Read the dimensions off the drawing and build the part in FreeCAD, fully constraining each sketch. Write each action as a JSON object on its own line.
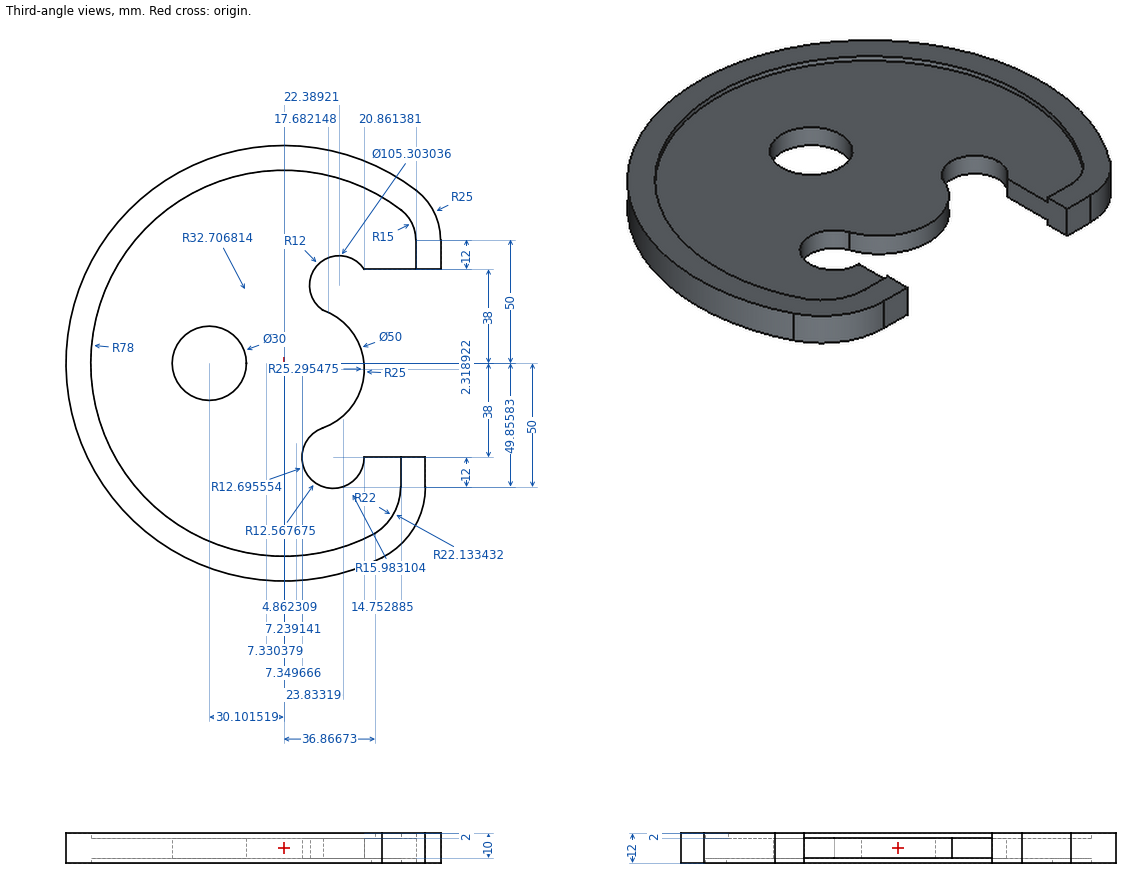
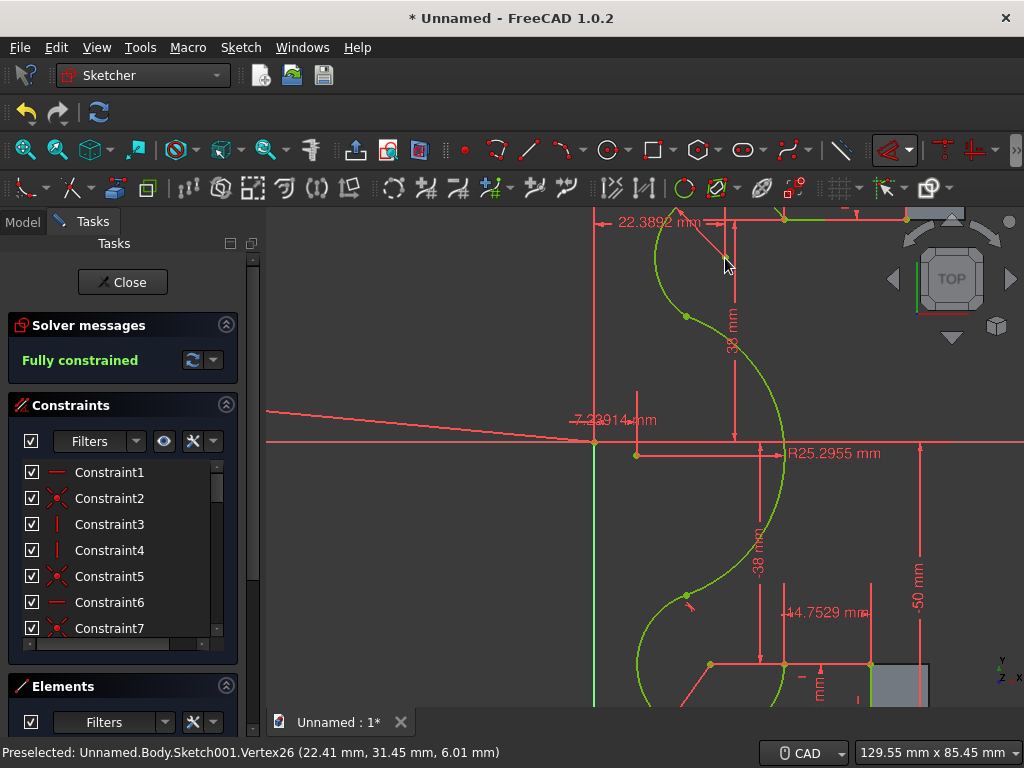
{"action": "left_click", "coordinate": [123, 282]}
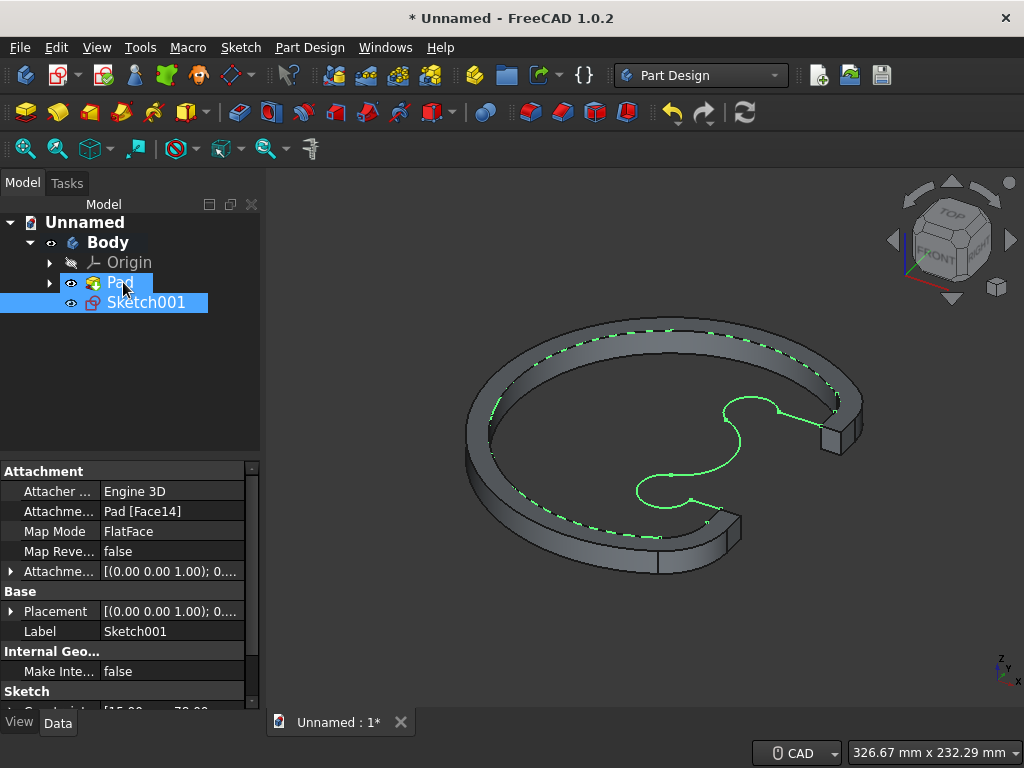
{"action": "left_click", "coordinate": [26, 112]}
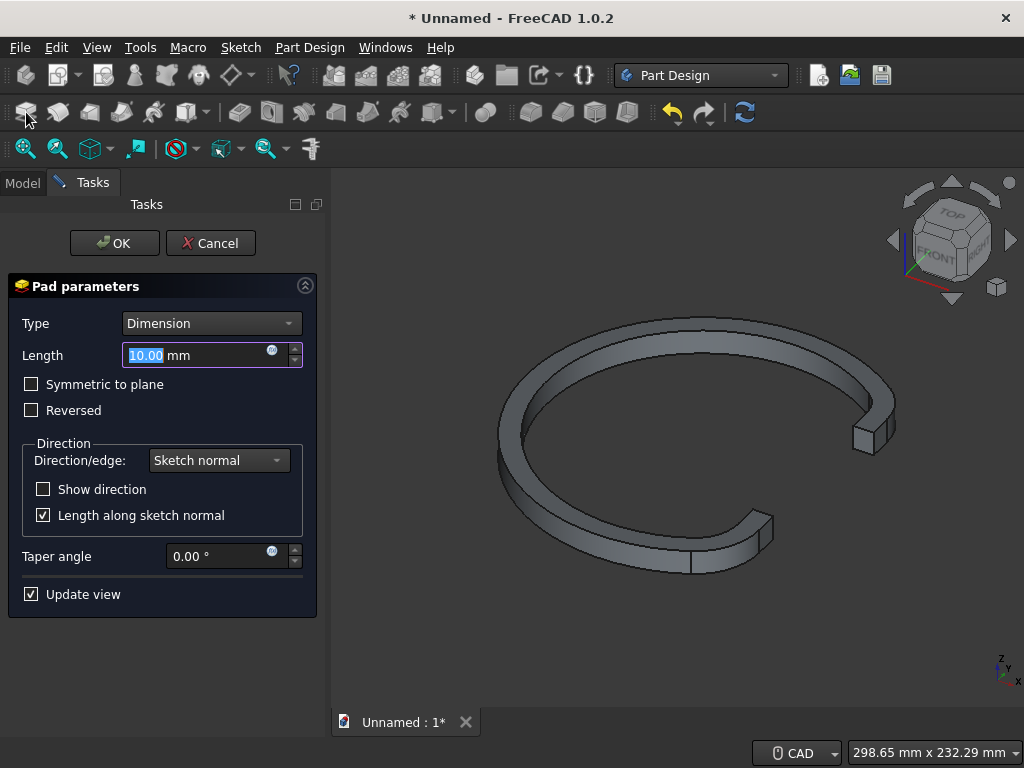
{"action": "type", "text": "10"}
{"action": "key", "text": "Tab"}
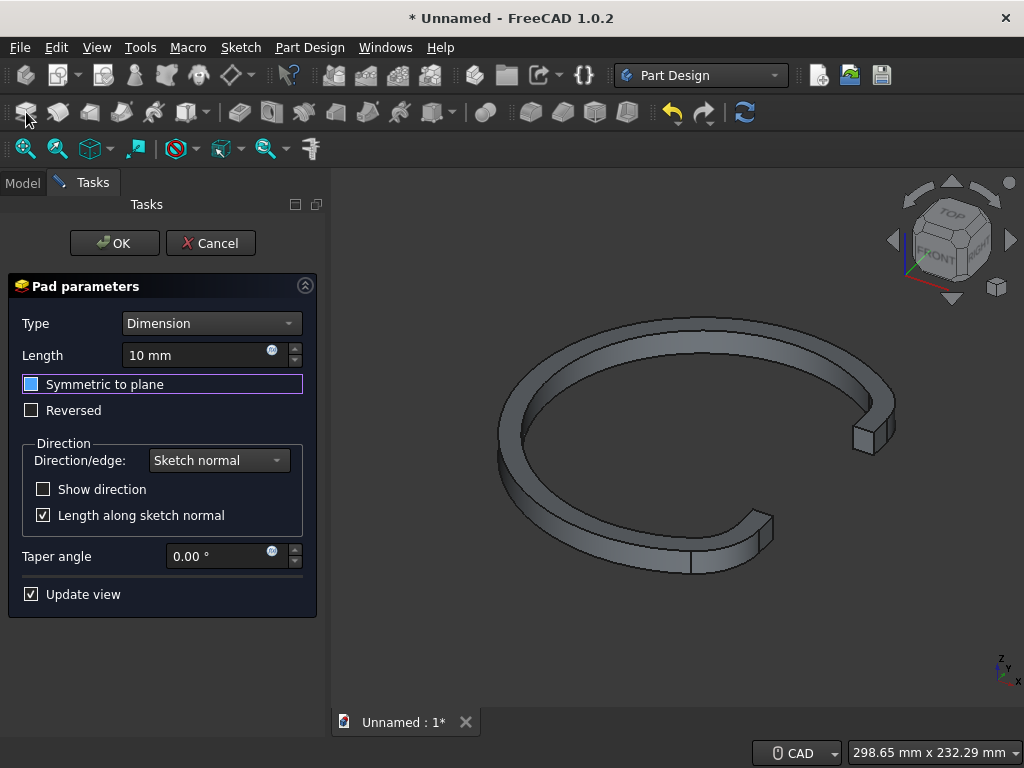
{"action": "left_click", "coordinate": [30, 410]}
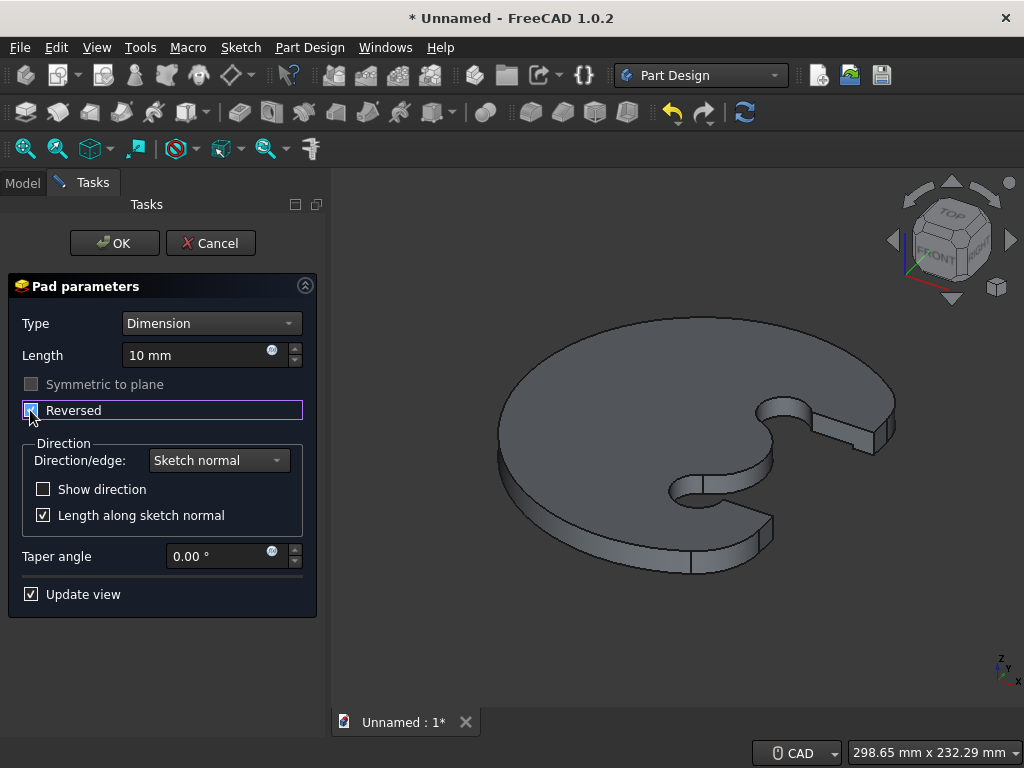
{"action": "left_click", "coordinate": [115, 243]}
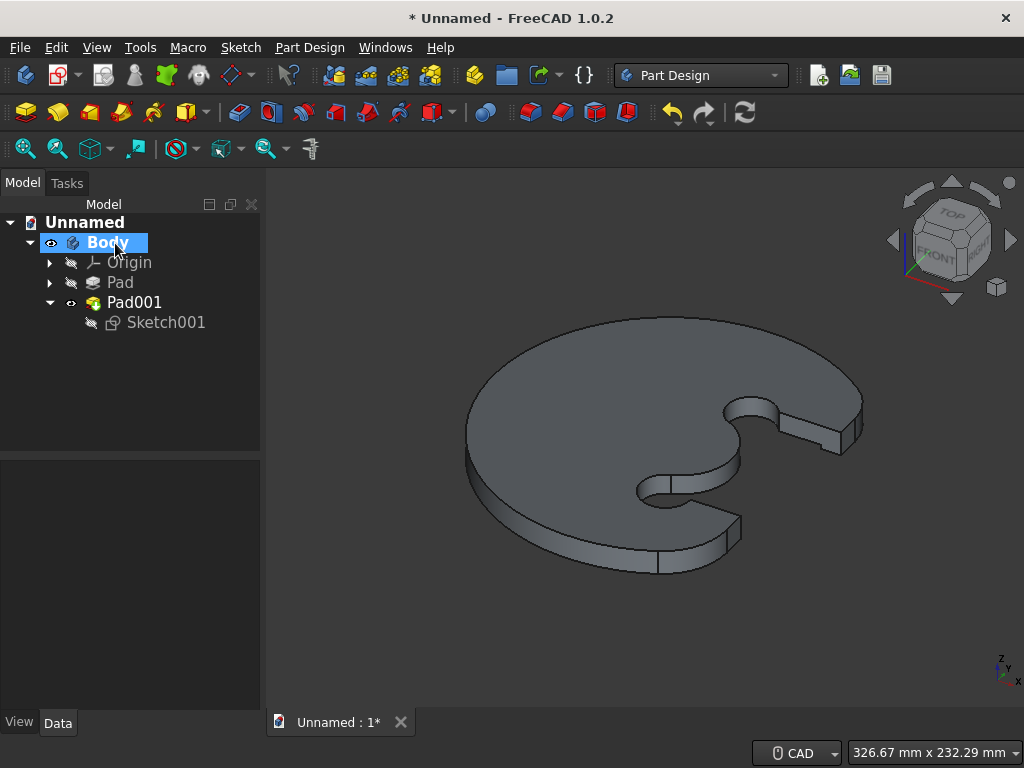
{"action": "left_click", "coordinate": [601, 411]}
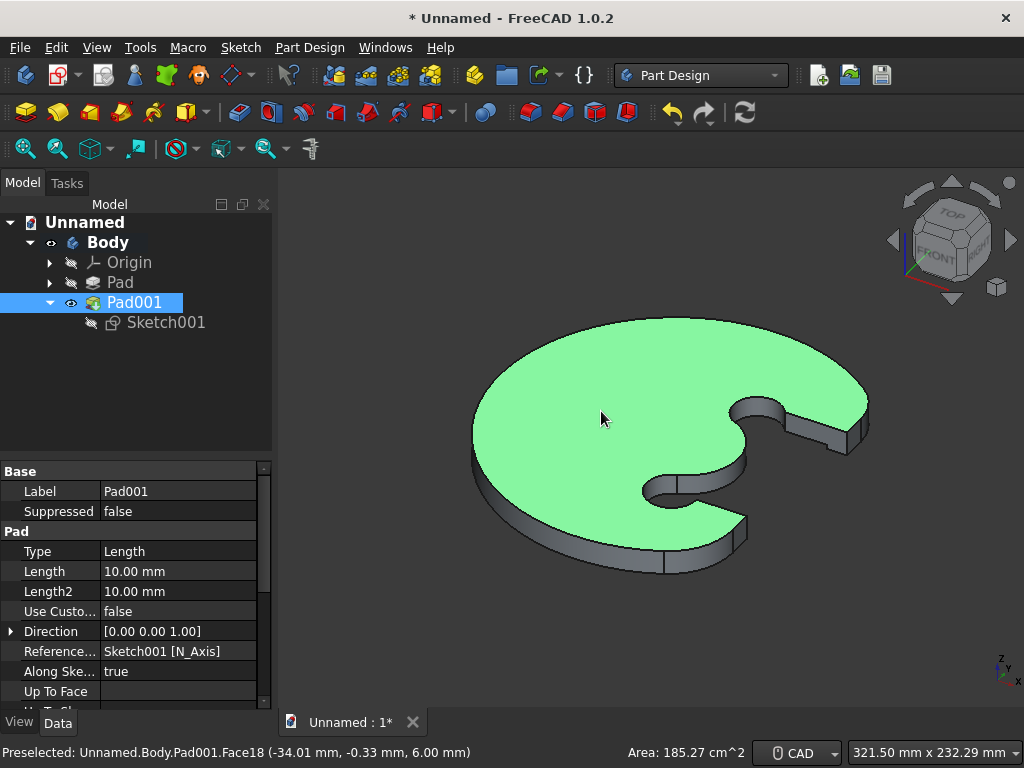
{"action": "left_click", "coordinate": [58, 76]}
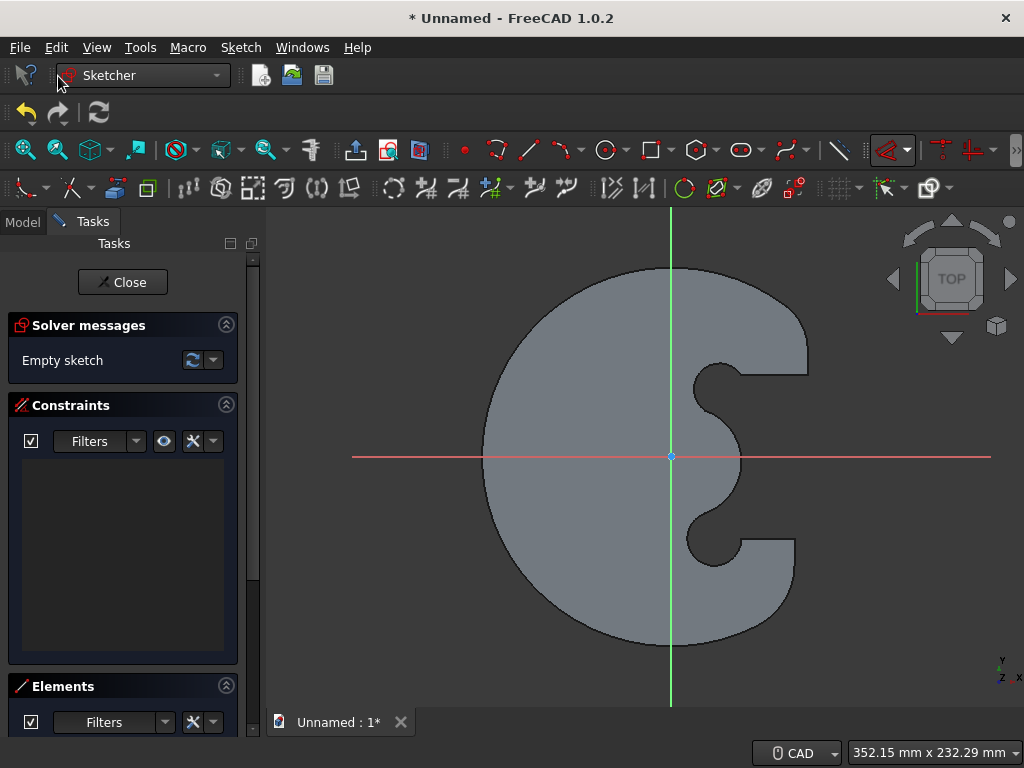
{"action": "key", "text": "g m"}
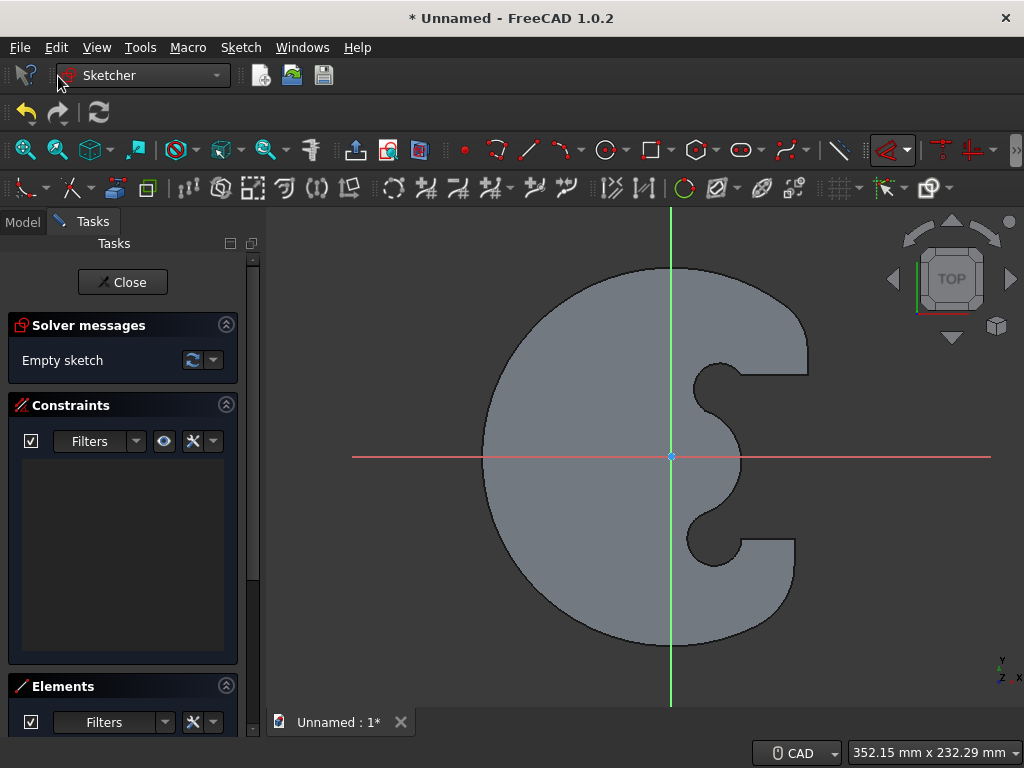
{"action": "left_click", "coordinate": [773, 565]}
{"action": "left_click", "coordinate": [773, 539]}
{"action": "left_click", "coordinate": [741, 539]}
{"action": "right_click", "coordinate": [741, 539]}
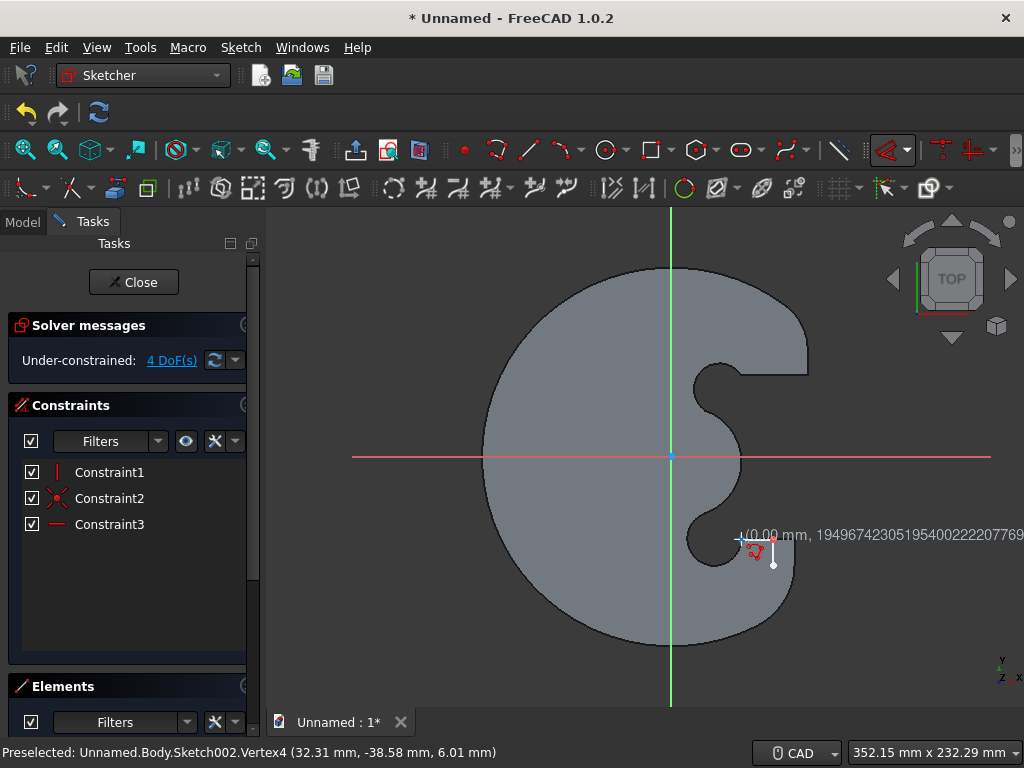
{"action": "left_click", "coordinate": [741, 375]}
{"action": "left_click", "coordinate": [786, 375]}
{"action": "left_click", "coordinate": [786, 349]}
{"action": "right_click", "coordinate": [786, 349]}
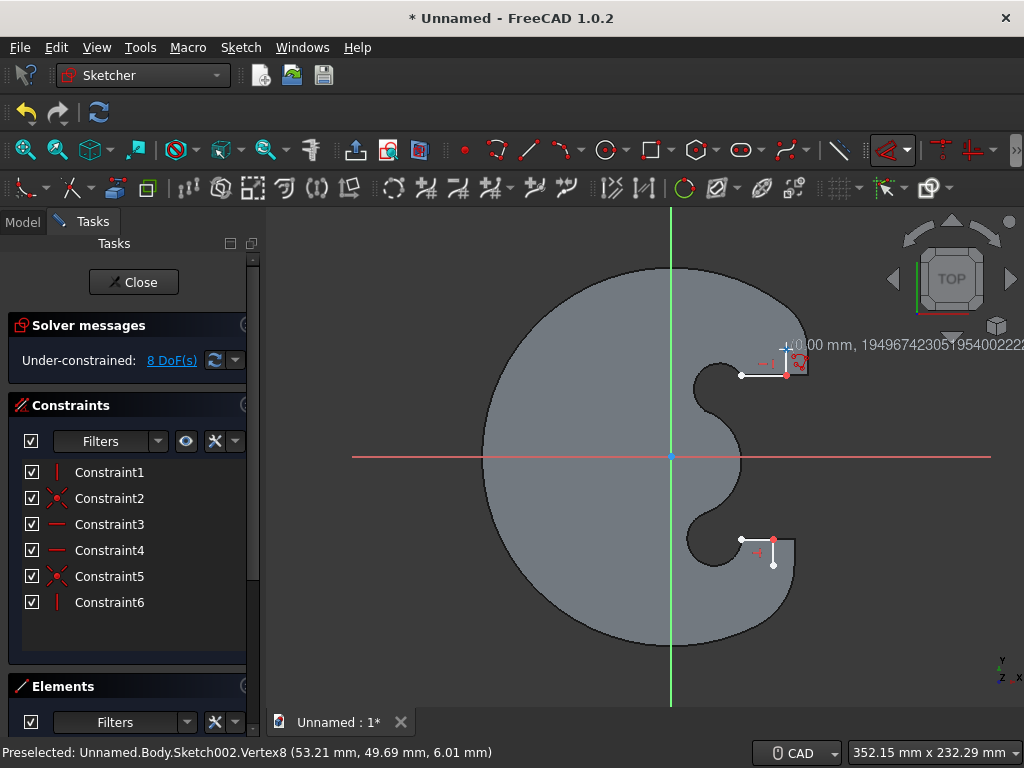
{"action": "key", "text": "g 3 a"}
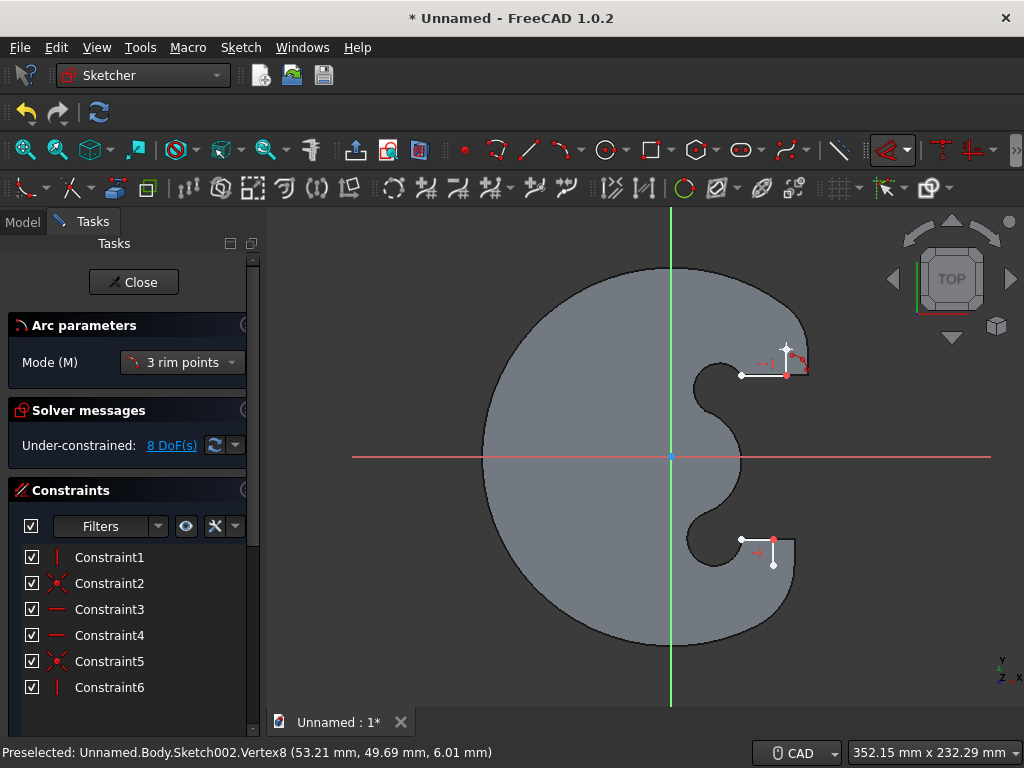
{"action": "left_click", "coordinate": [741, 540]}
{"action": "left_click", "coordinate": [723, 564]}